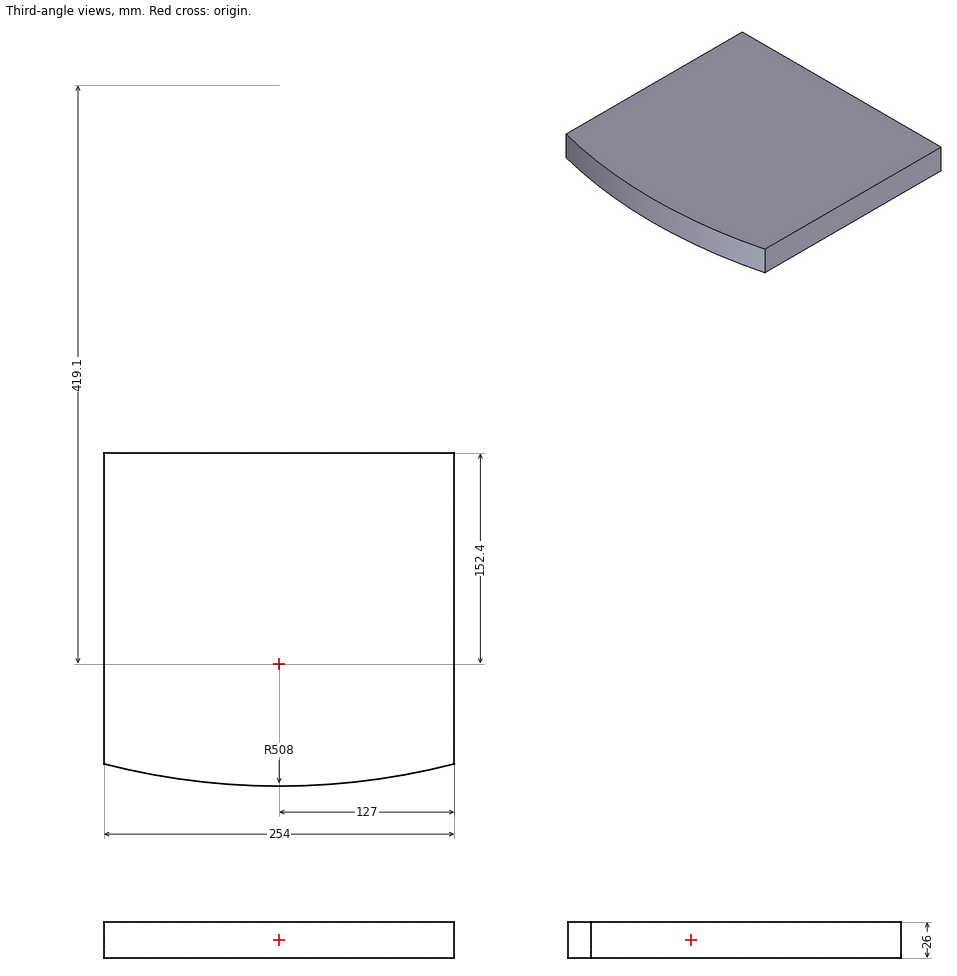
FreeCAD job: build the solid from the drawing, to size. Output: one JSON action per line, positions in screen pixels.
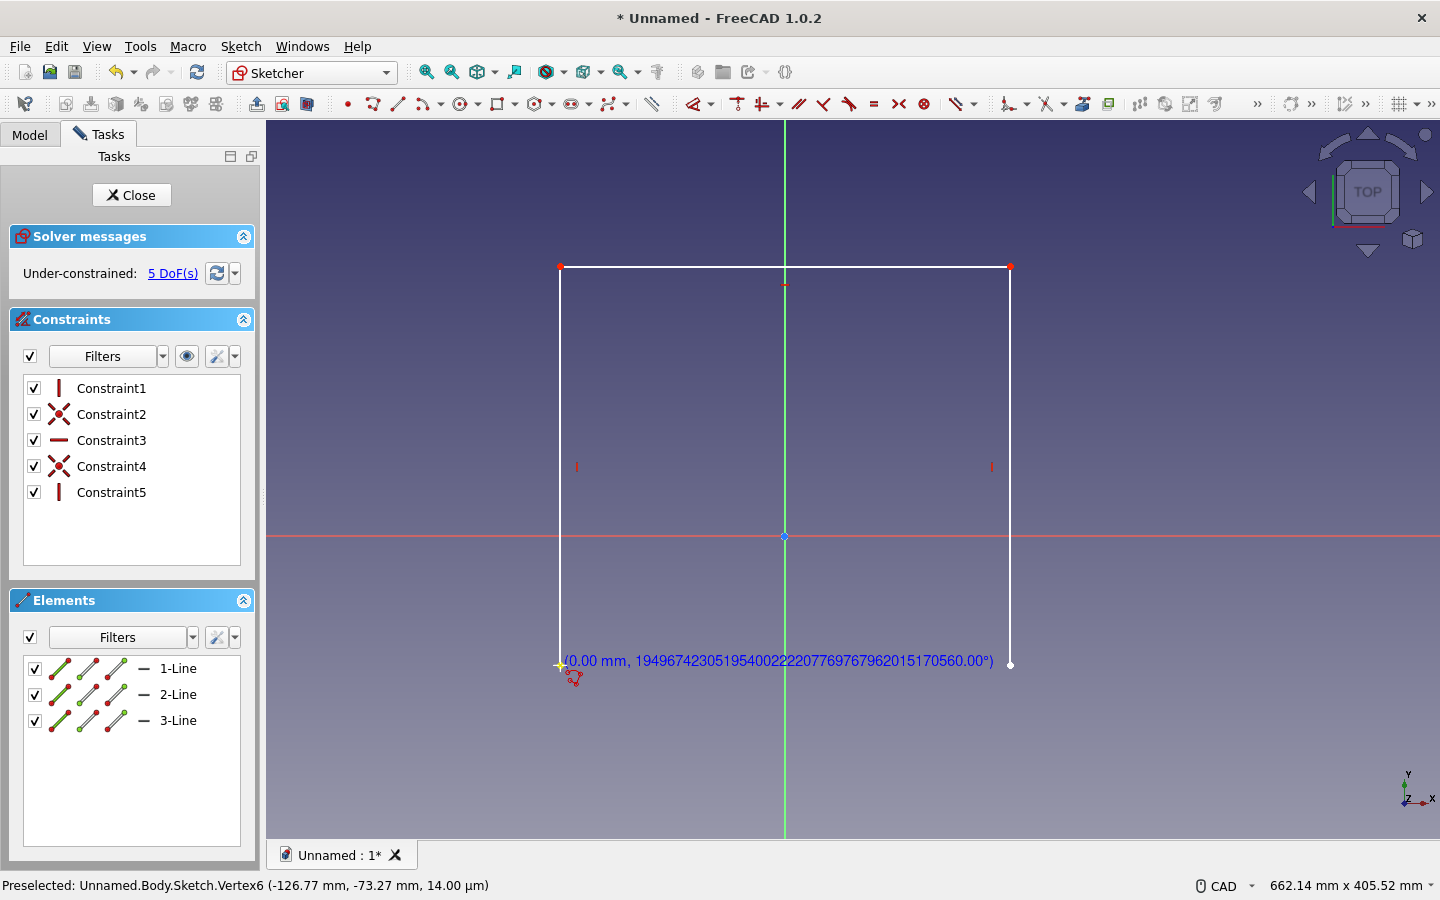
{"action": "key", "text": "g 3 a"}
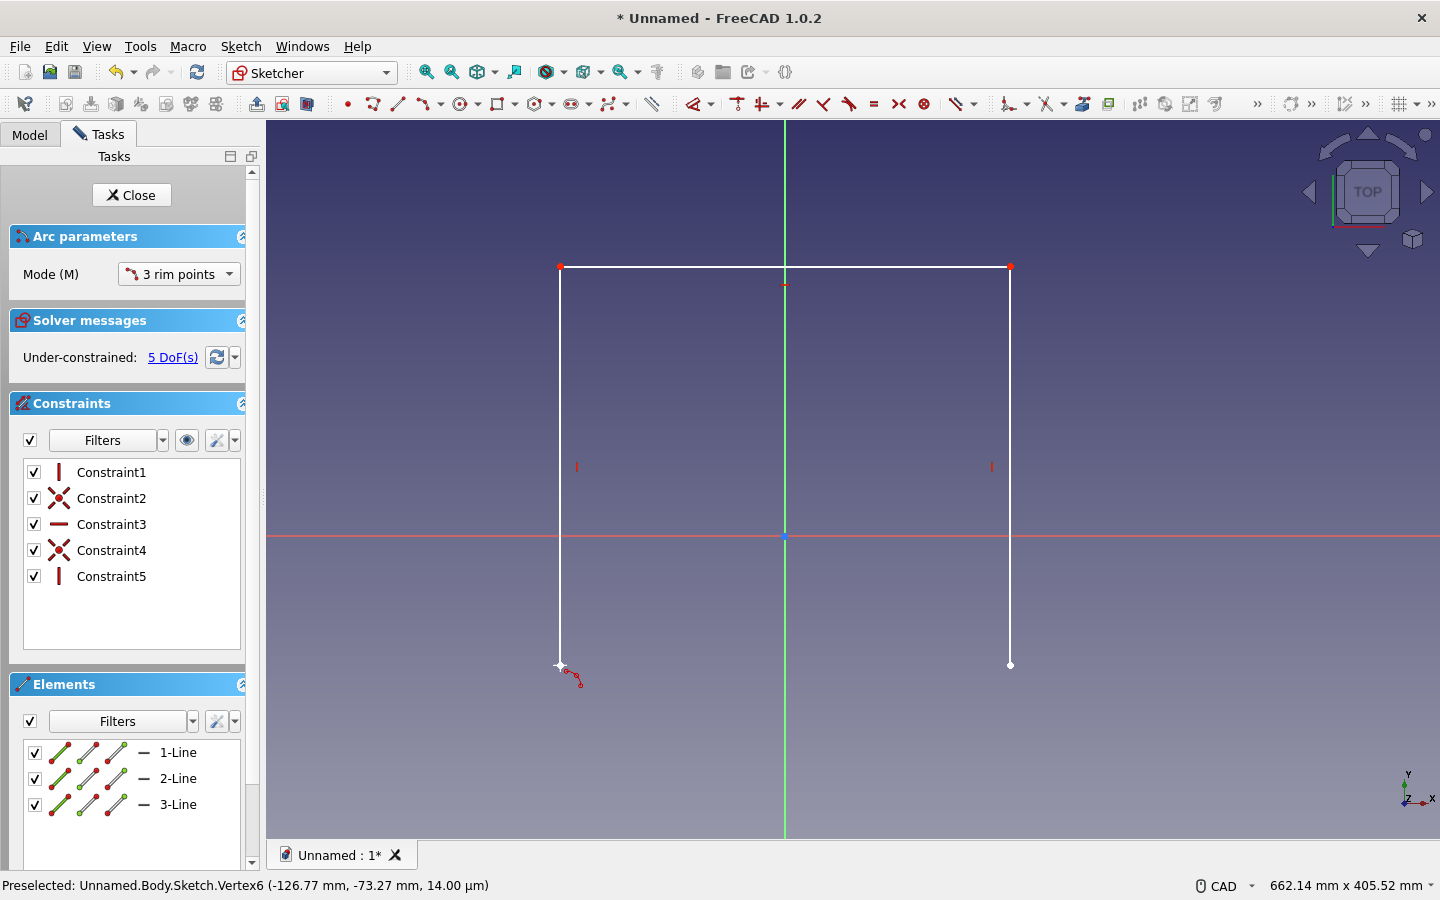
{"action": "left_click", "coordinate": [560, 666]}
{"action": "left_click", "coordinate": [1010, 666]}
{"action": "left_click", "coordinate": [739, 693]}
{"action": "key", "text": "Escape"}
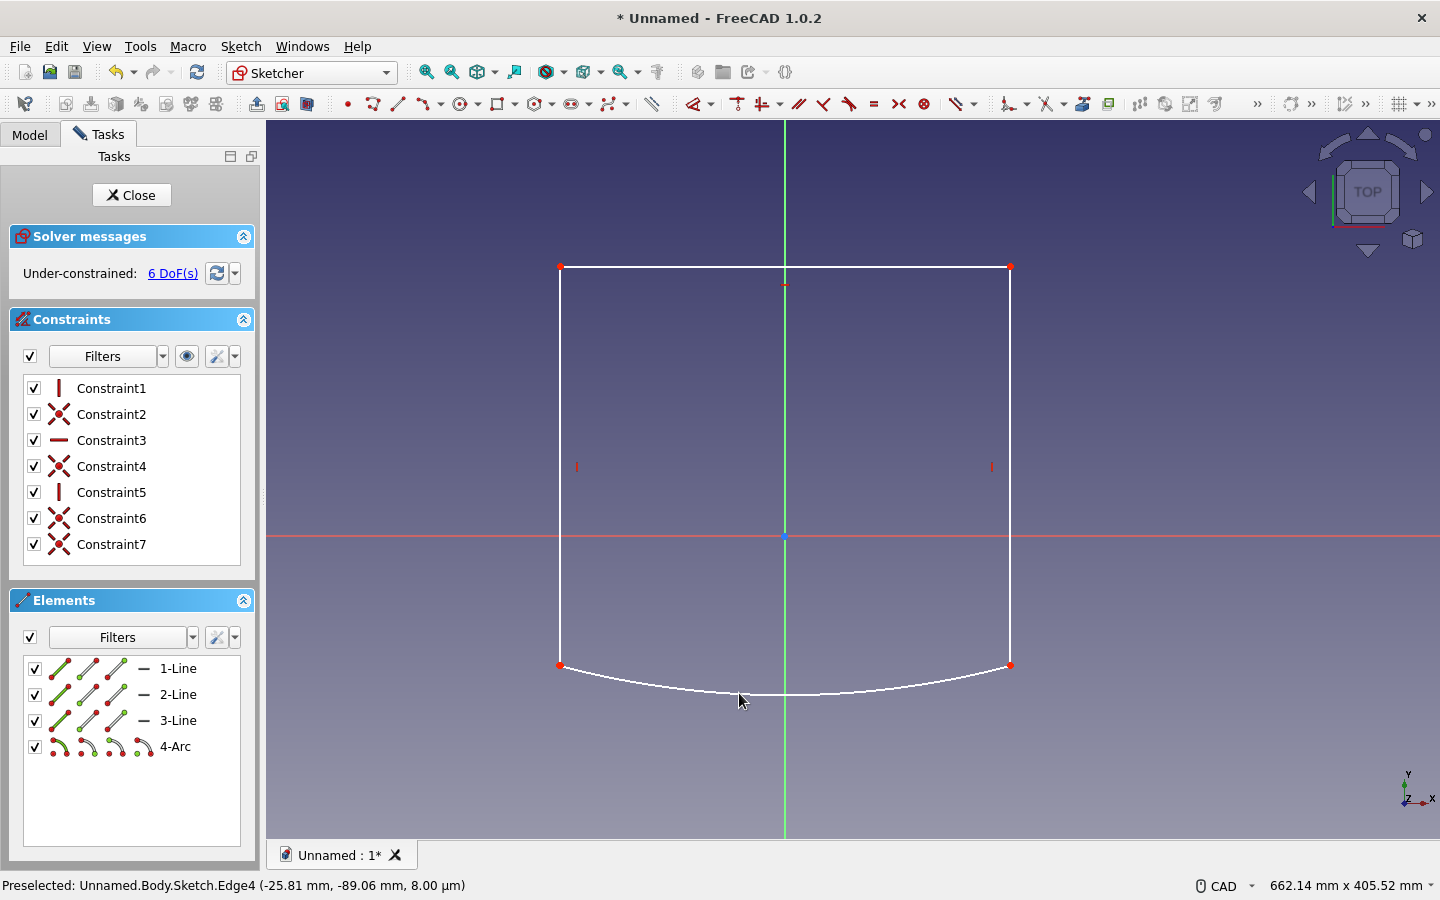
{"action": "scroll", "coordinate": [784, 754], "scroll_direction": "down", "scroll_amount": 3}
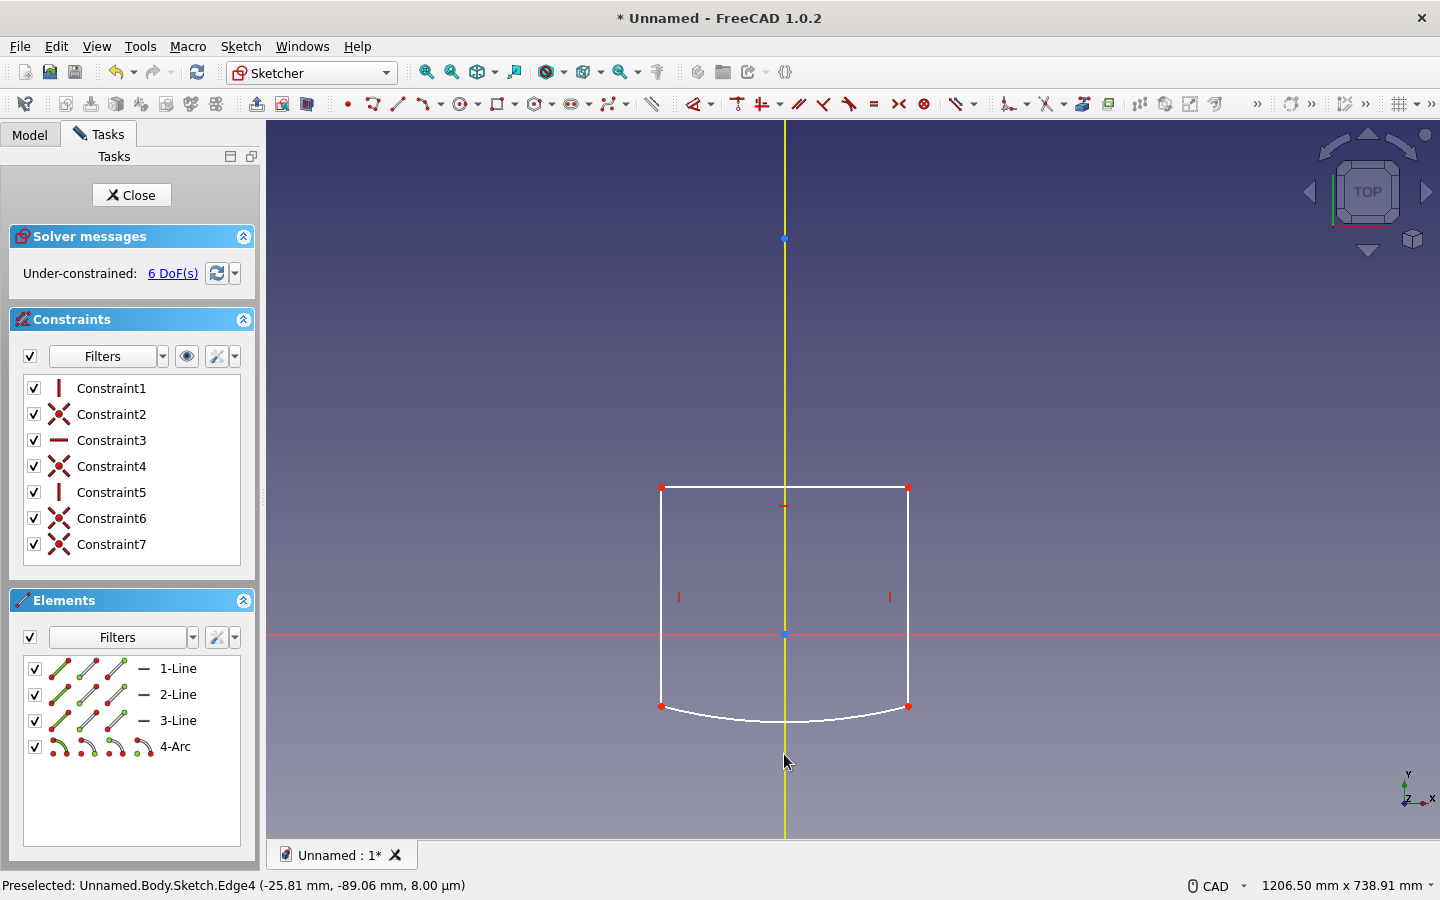
{"action": "left_click", "coordinate": [785, 238]}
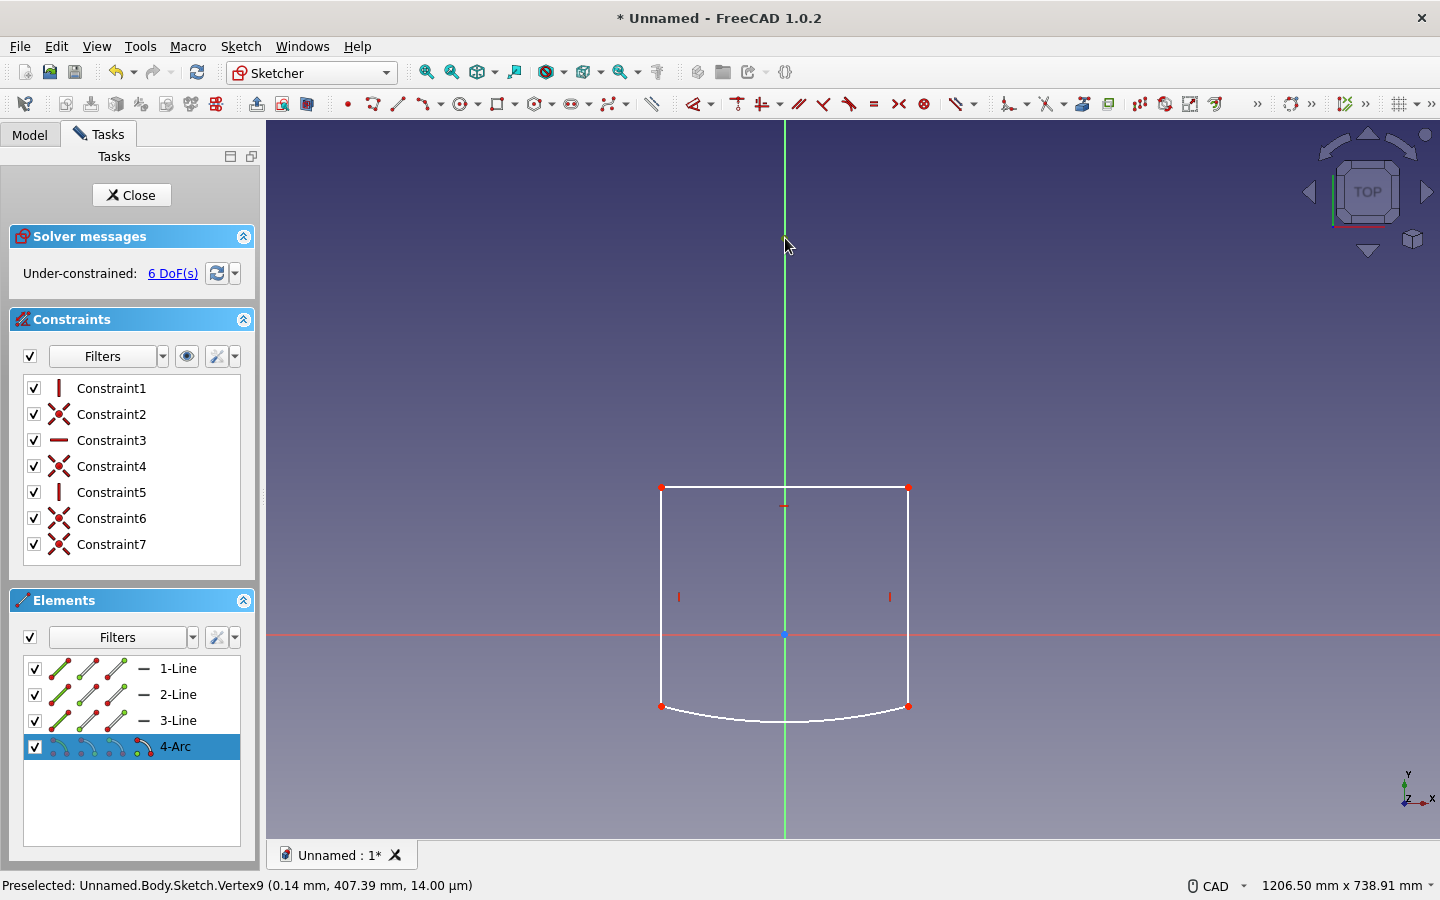
{"action": "left_click", "coordinate": [785, 764]}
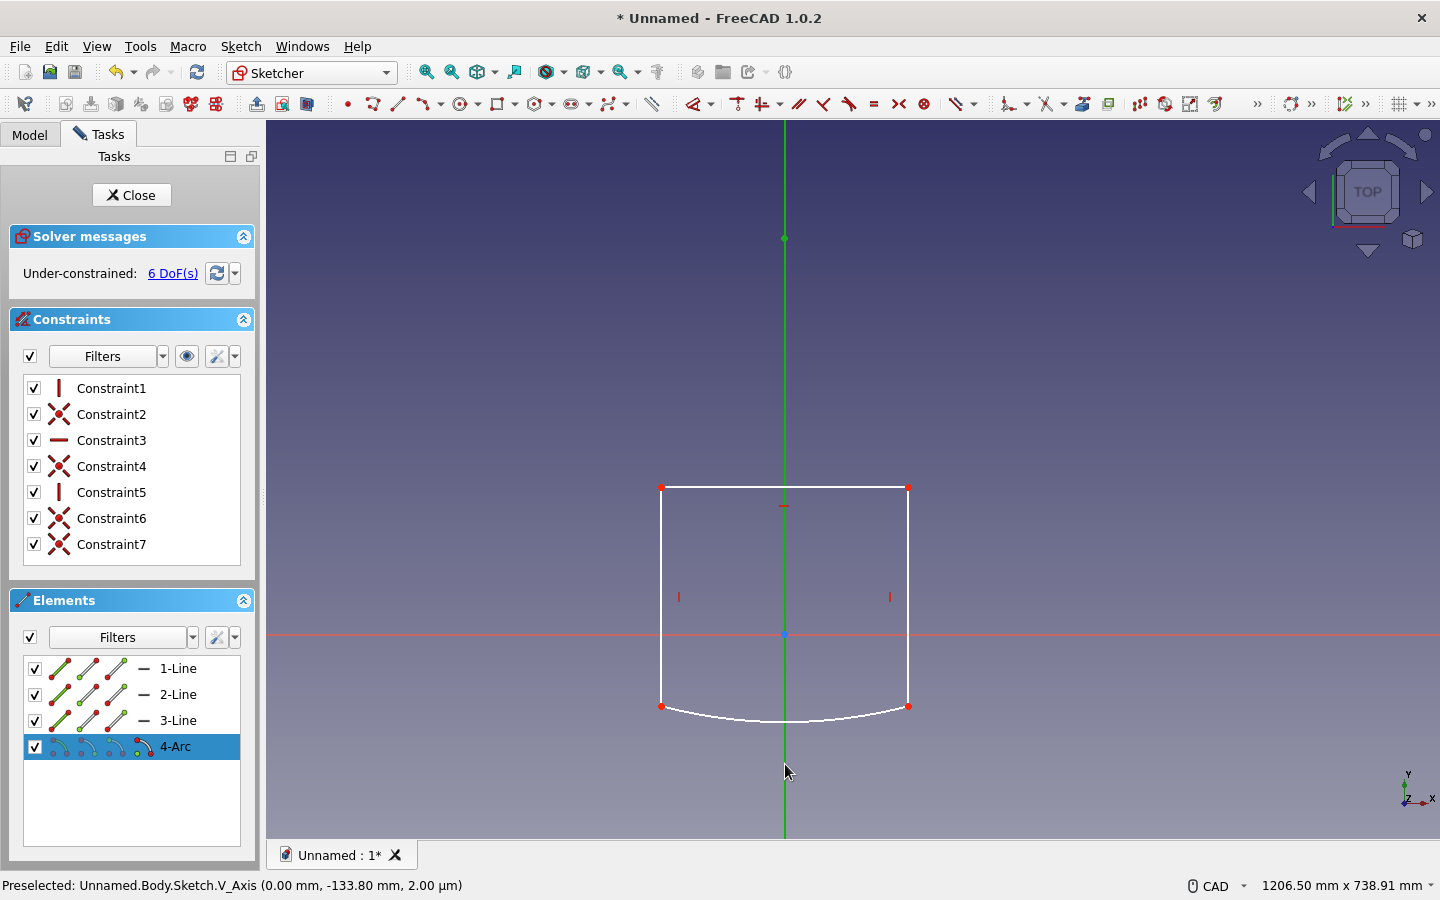
{"action": "left_click", "coordinate": [737, 104]}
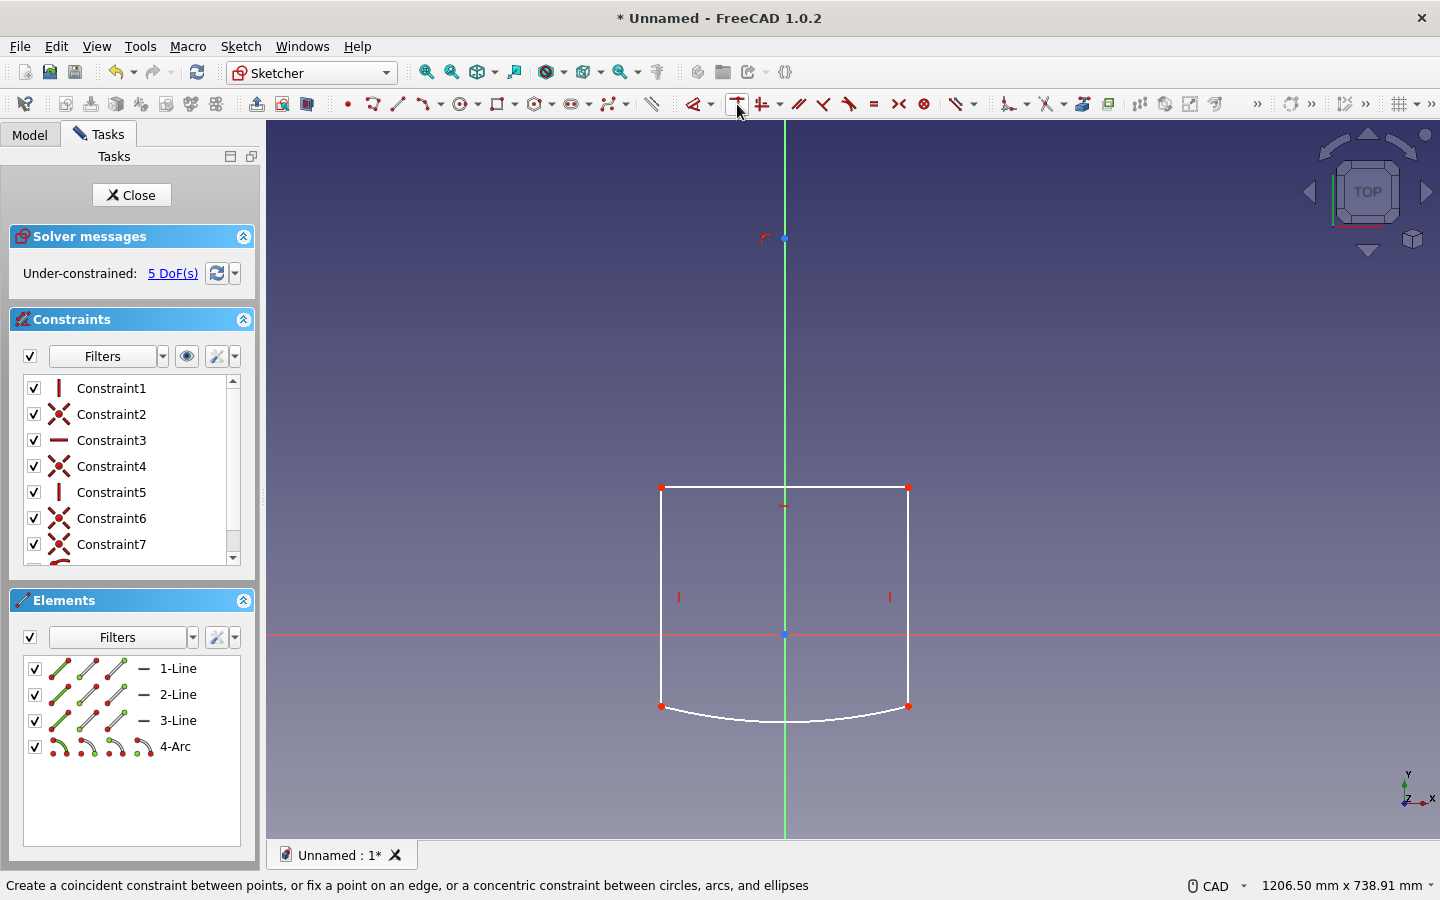
{"action": "left_click", "coordinate": [692, 104]}